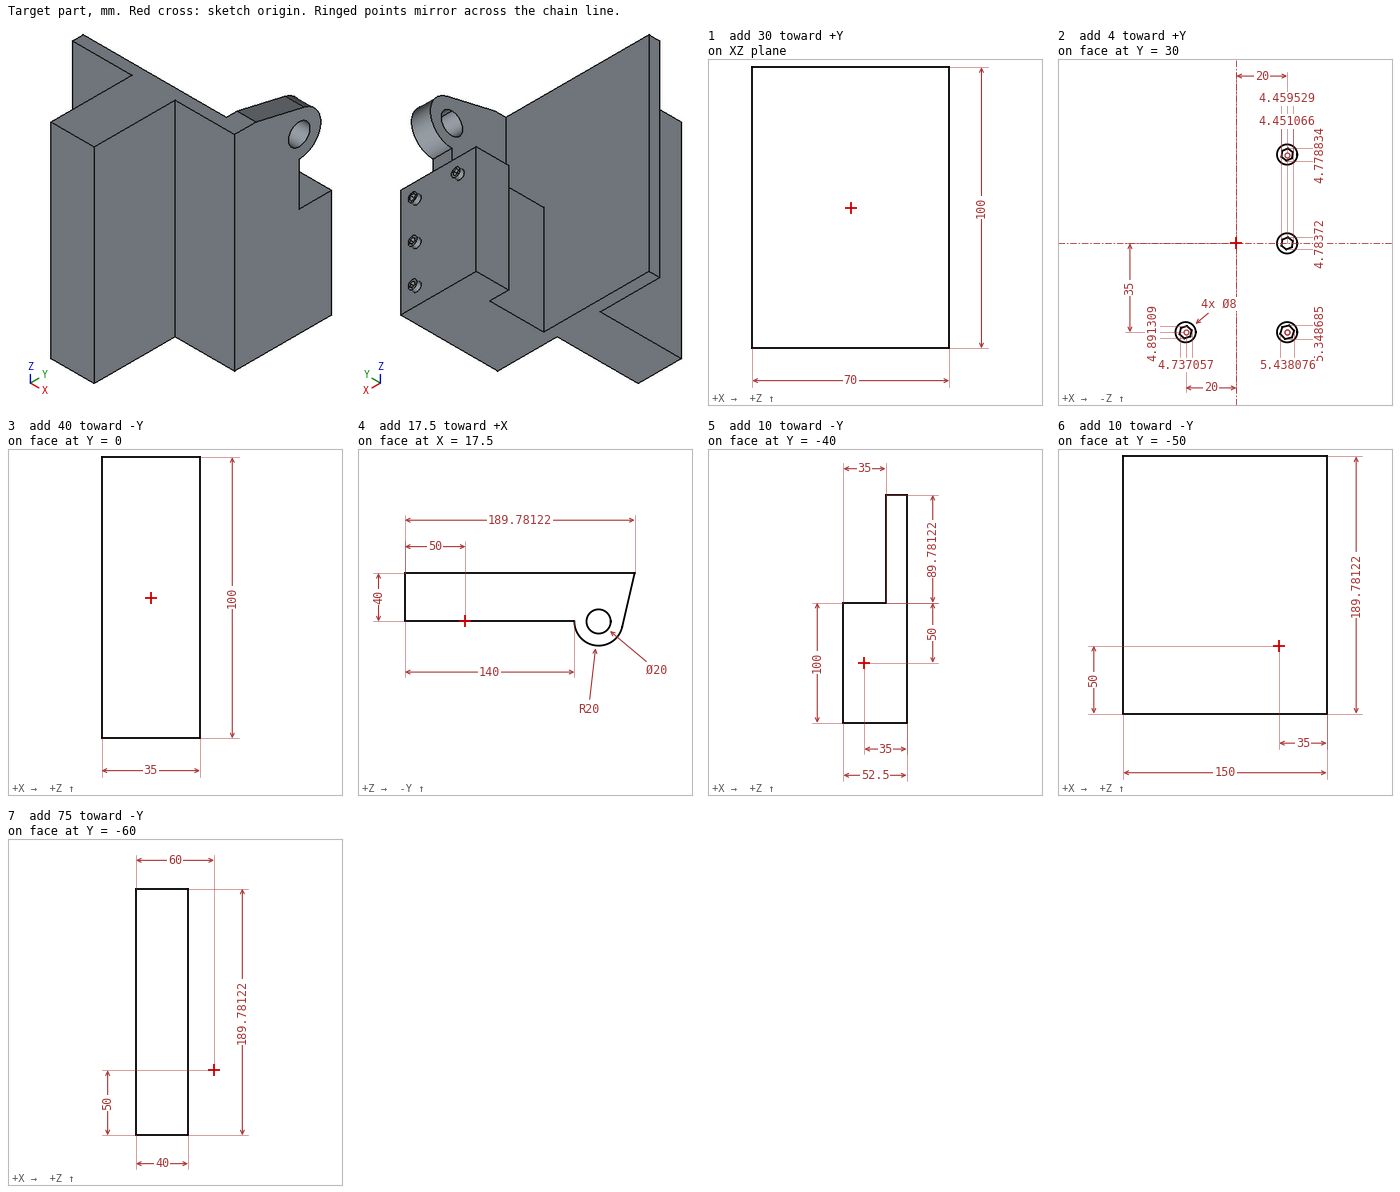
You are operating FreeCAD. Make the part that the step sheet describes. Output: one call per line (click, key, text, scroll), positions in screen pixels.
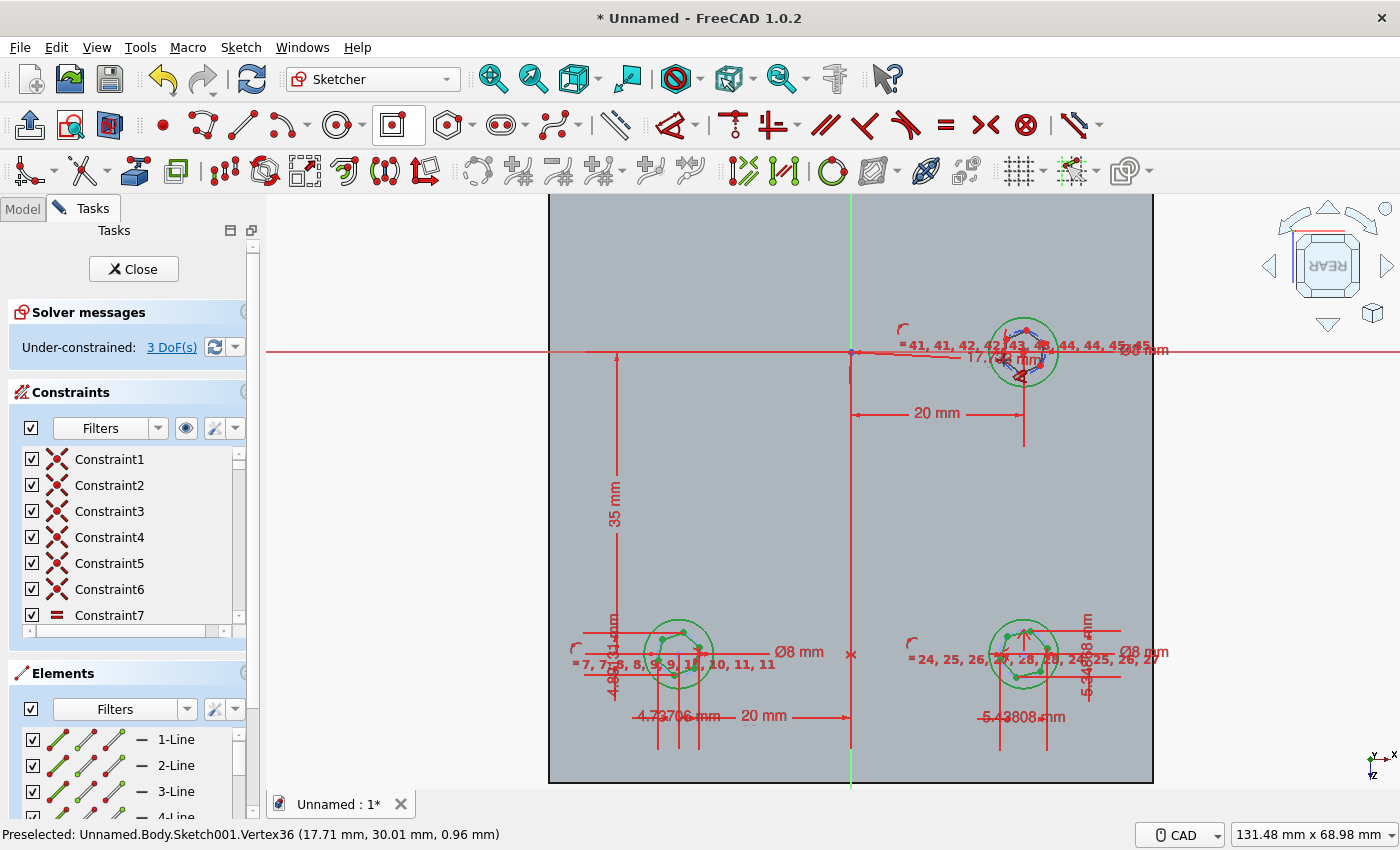
click(1044, 344)
click(1024, 418)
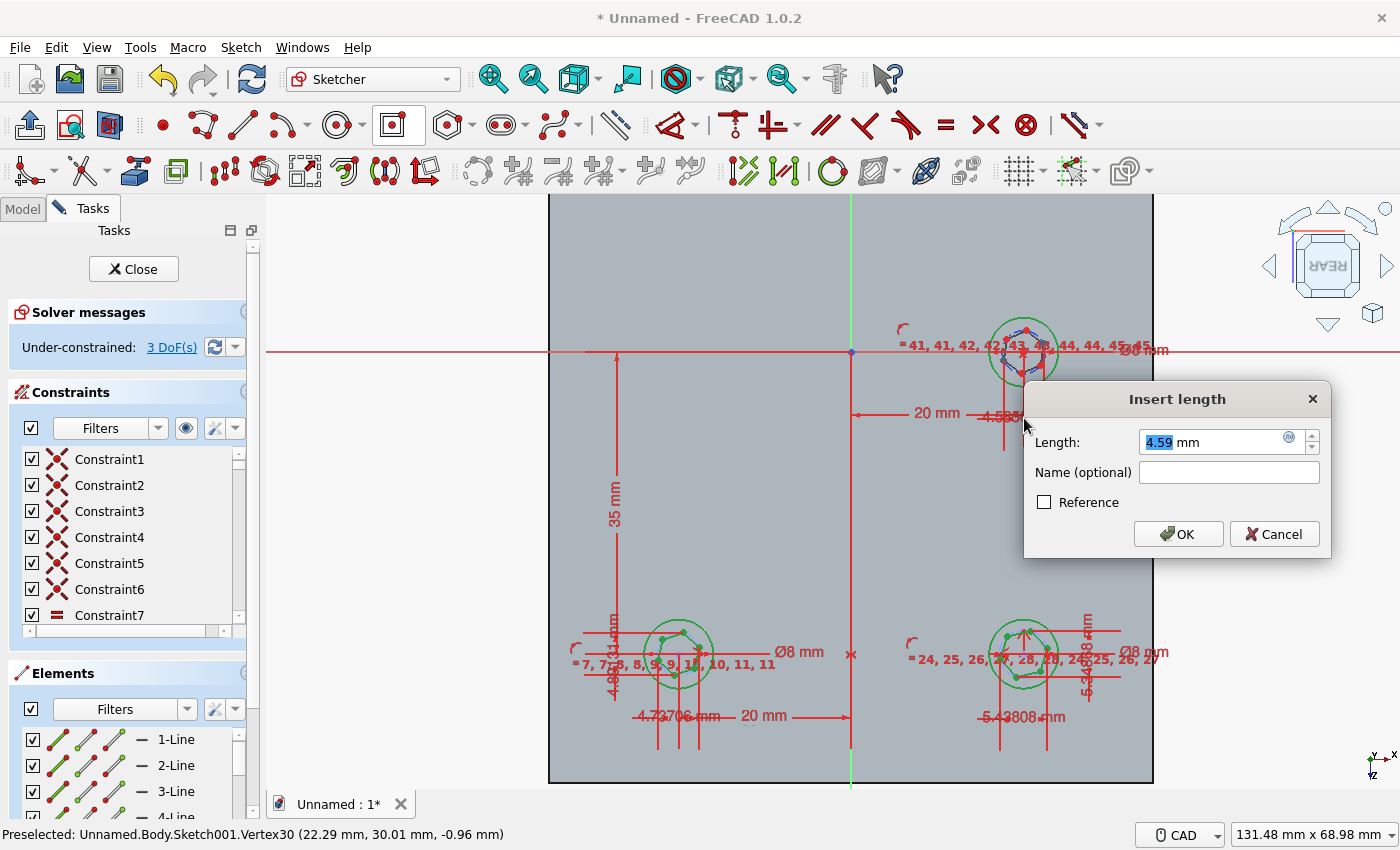
text(4.459529)
key(Return)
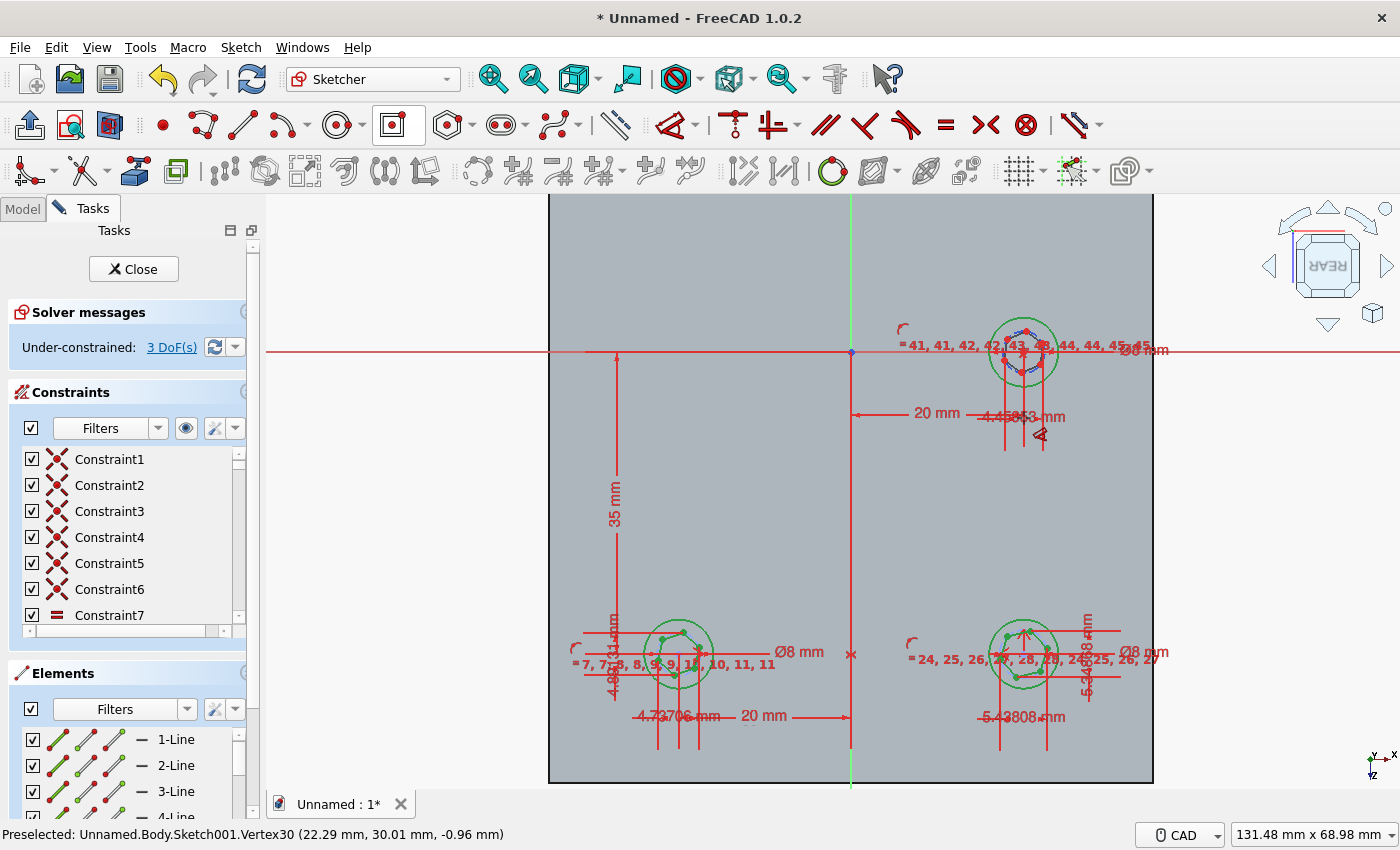
click(1021, 373)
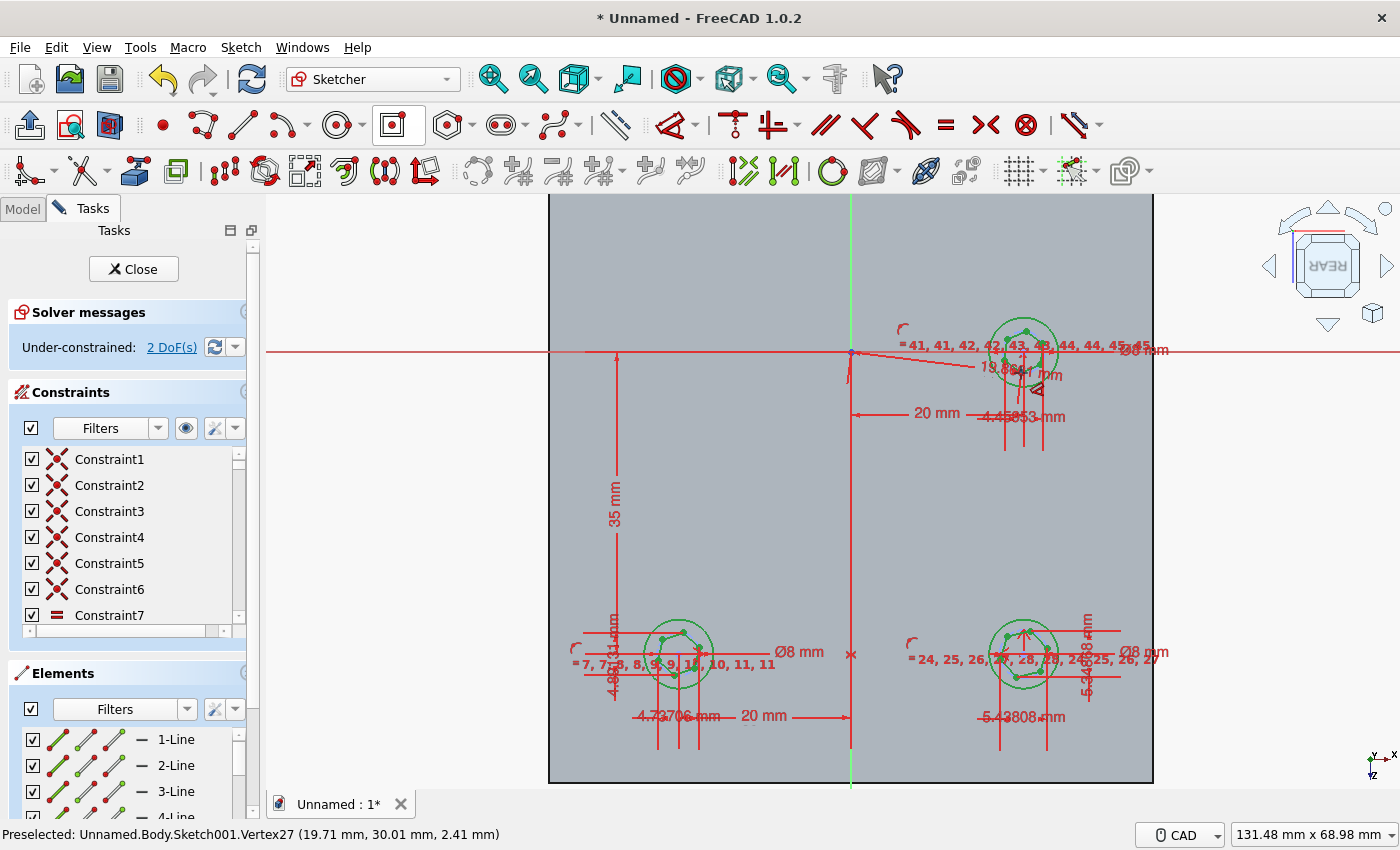
click(1026, 331)
click(1084, 338)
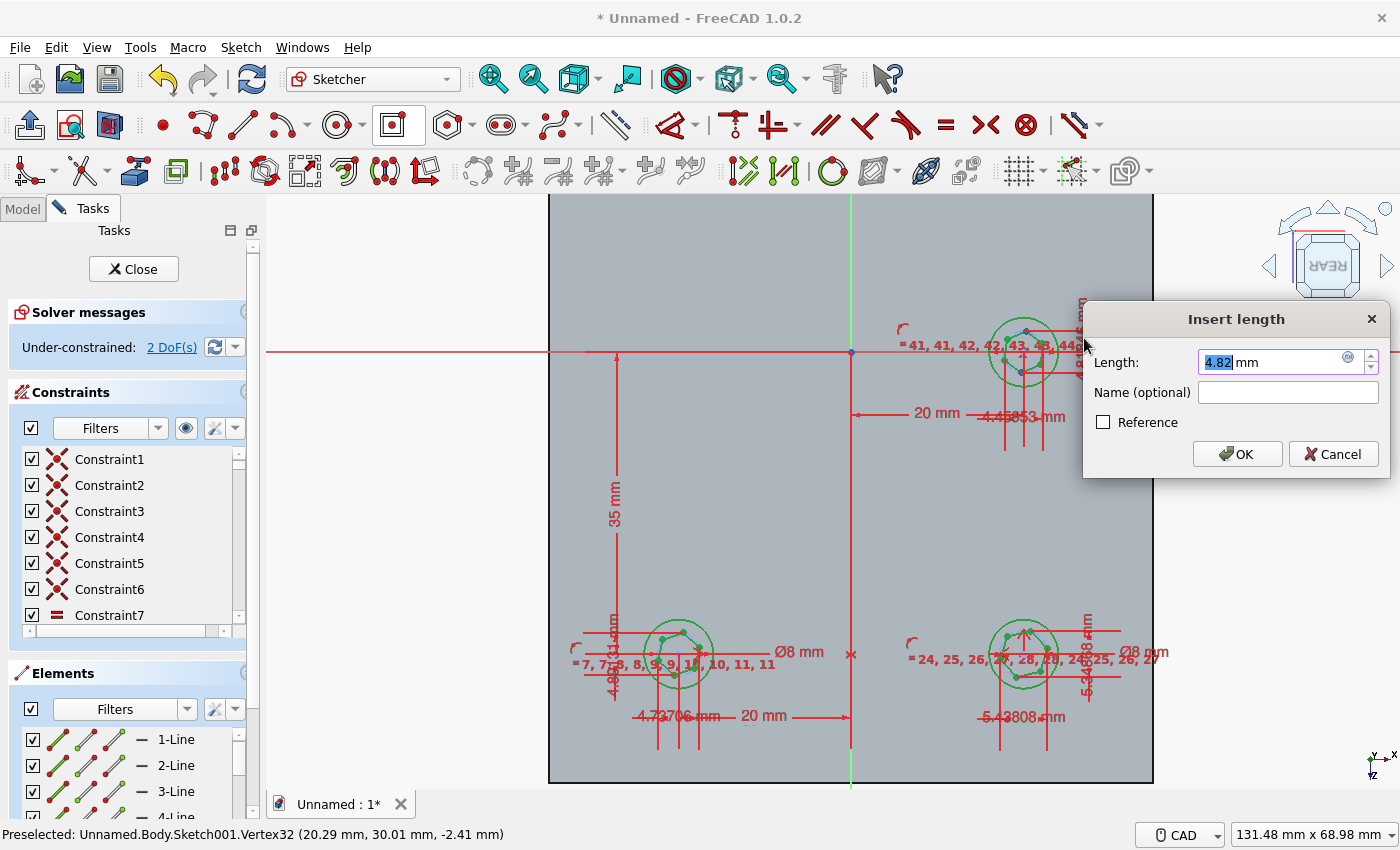
text(4.78372)
key(Return)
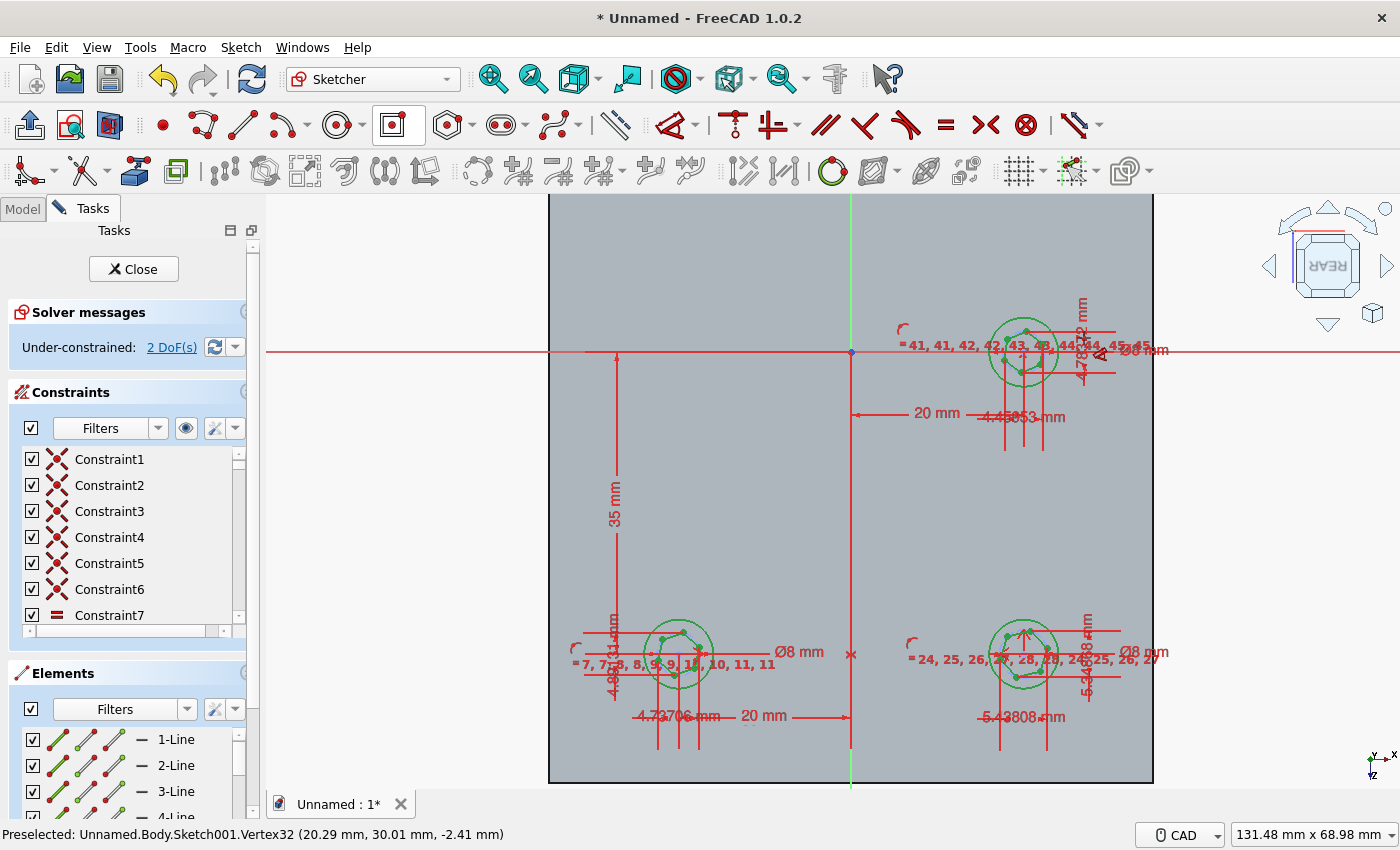
scroll(659, 661, down, 3)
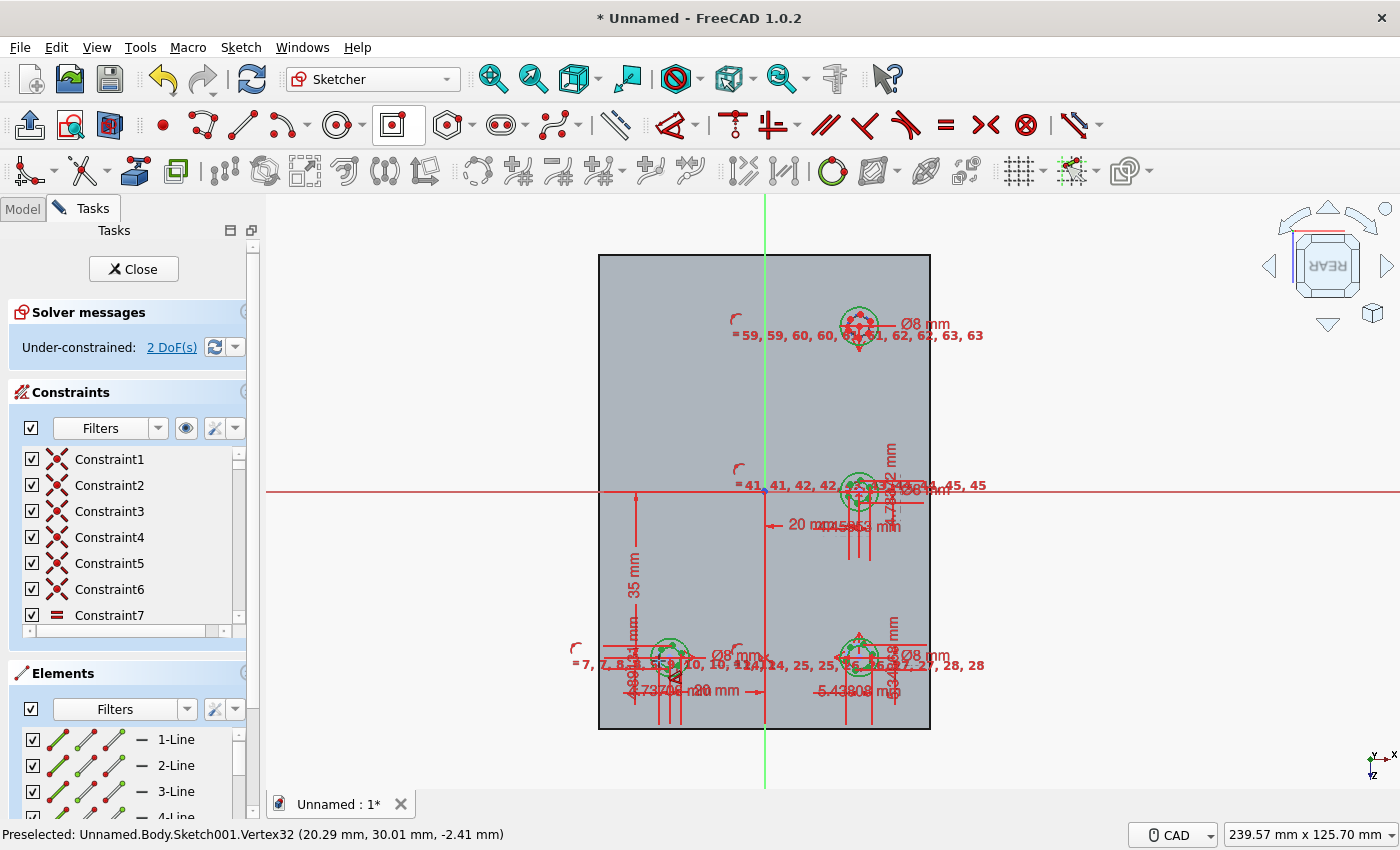
scroll(849, 331, up, 4)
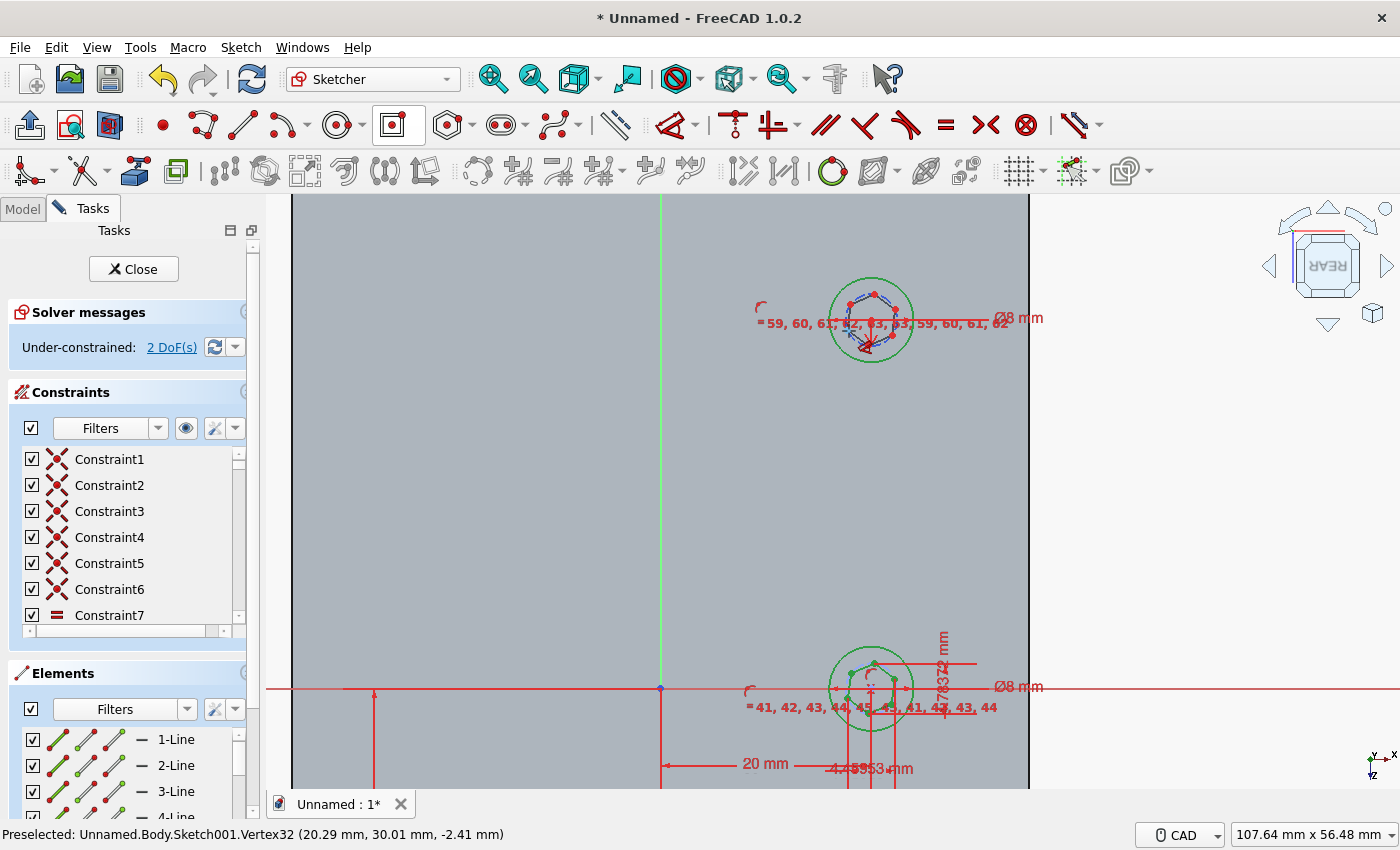
click(848, 330)